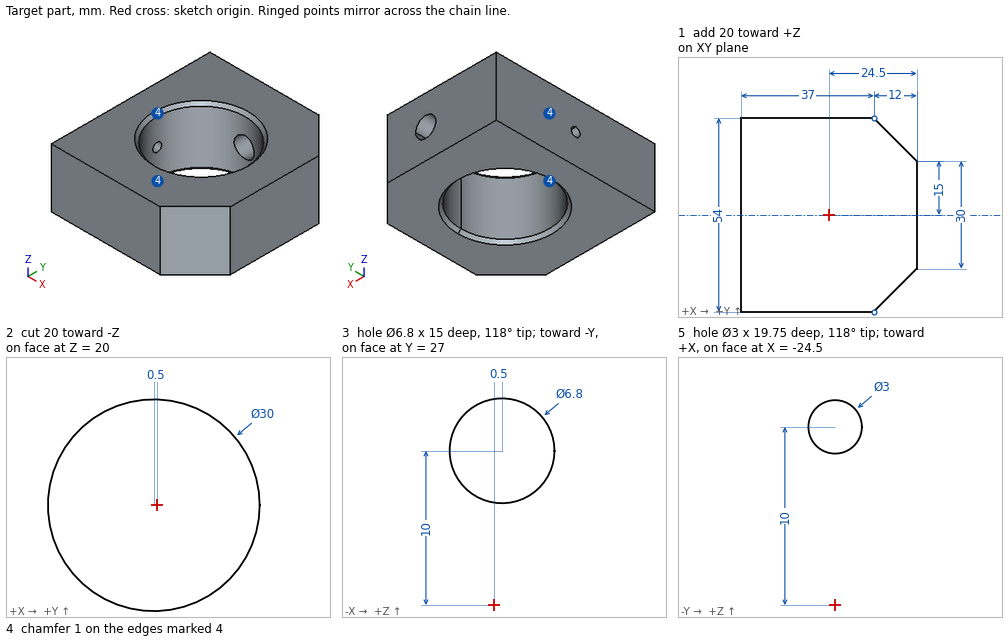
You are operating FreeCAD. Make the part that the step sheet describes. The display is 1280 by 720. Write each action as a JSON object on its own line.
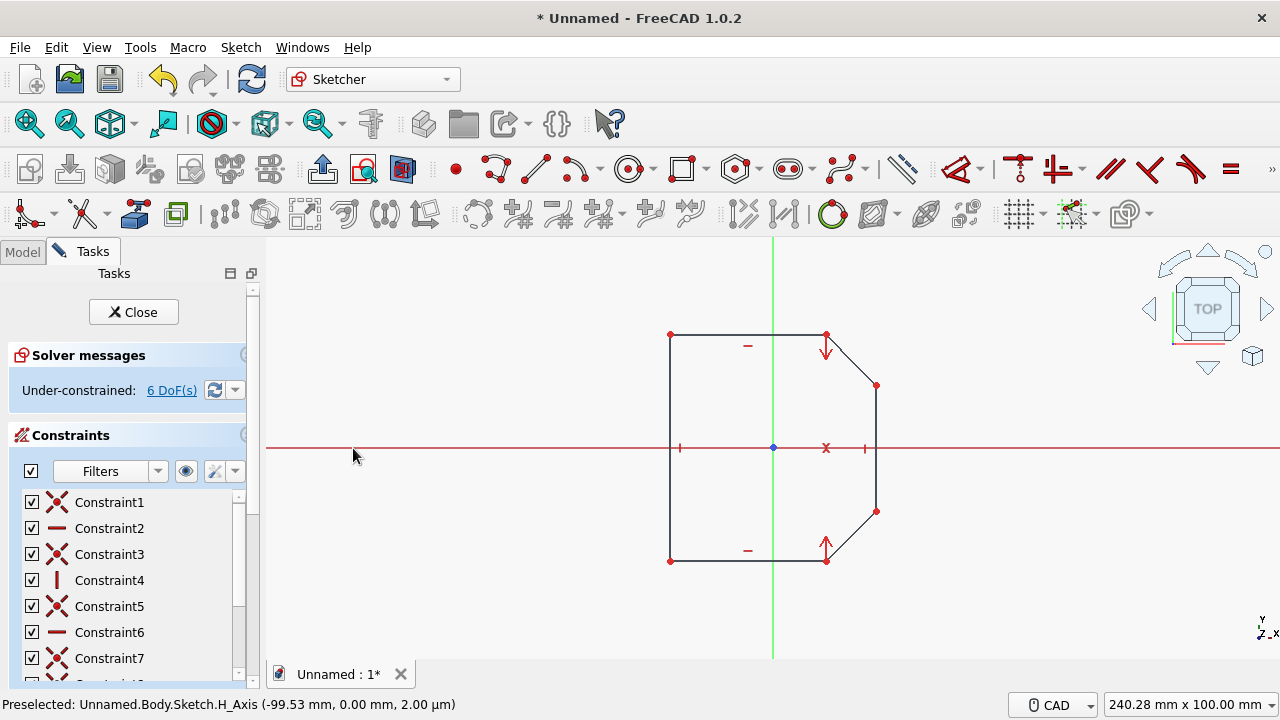
{"action": "left_click", "coordinate": [717, 335]}
{"action": "left_click", "coordinate": [748, 301]}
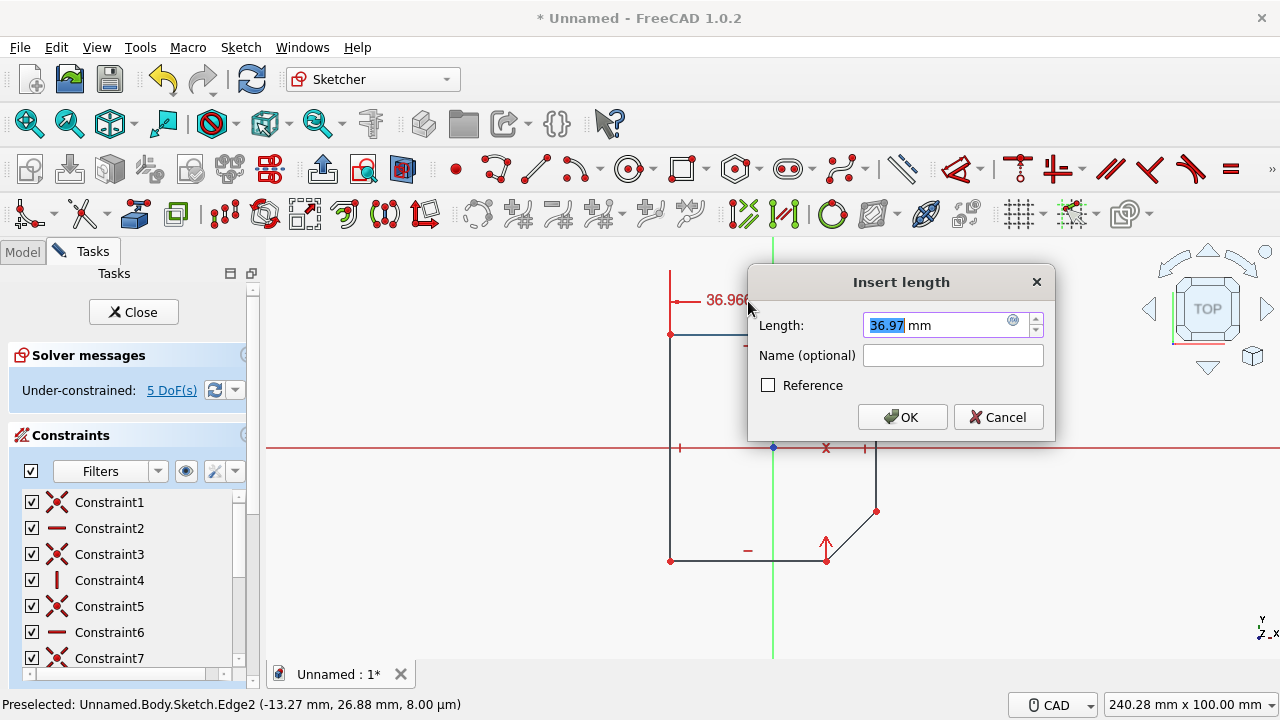
{"action": "type", "text": "37"}
{"action": "key", "text": "Return"}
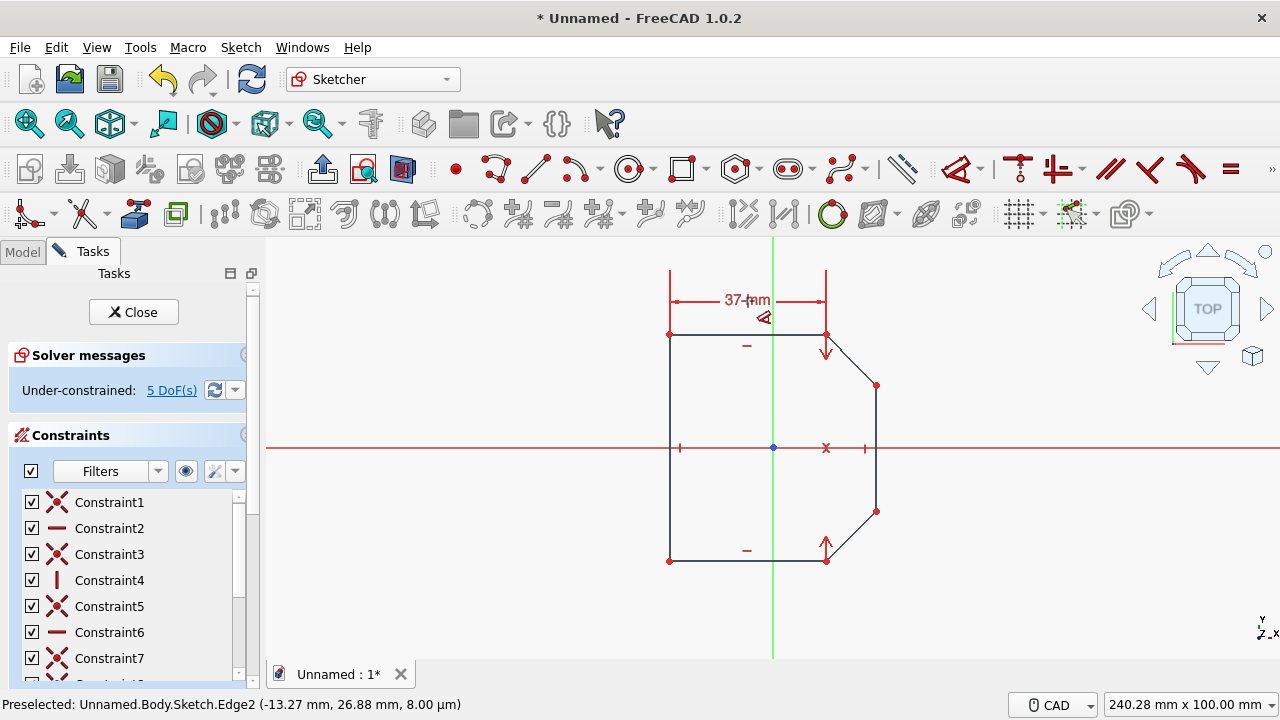
{"action": "left_click", "coordinate": [670, 403]}
{"action": "left_click", "coordinate": [636, 396]}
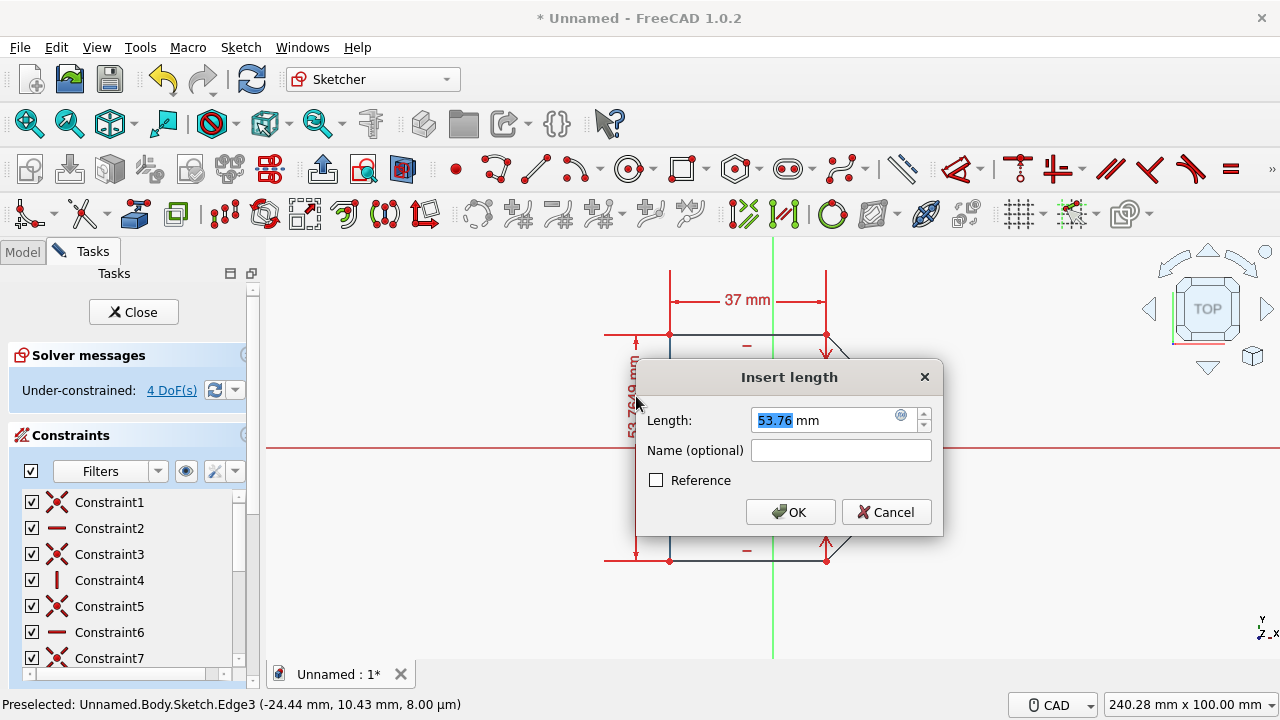
{"action": "type", "text": "54"}
{"action": "key", "text": "Return"}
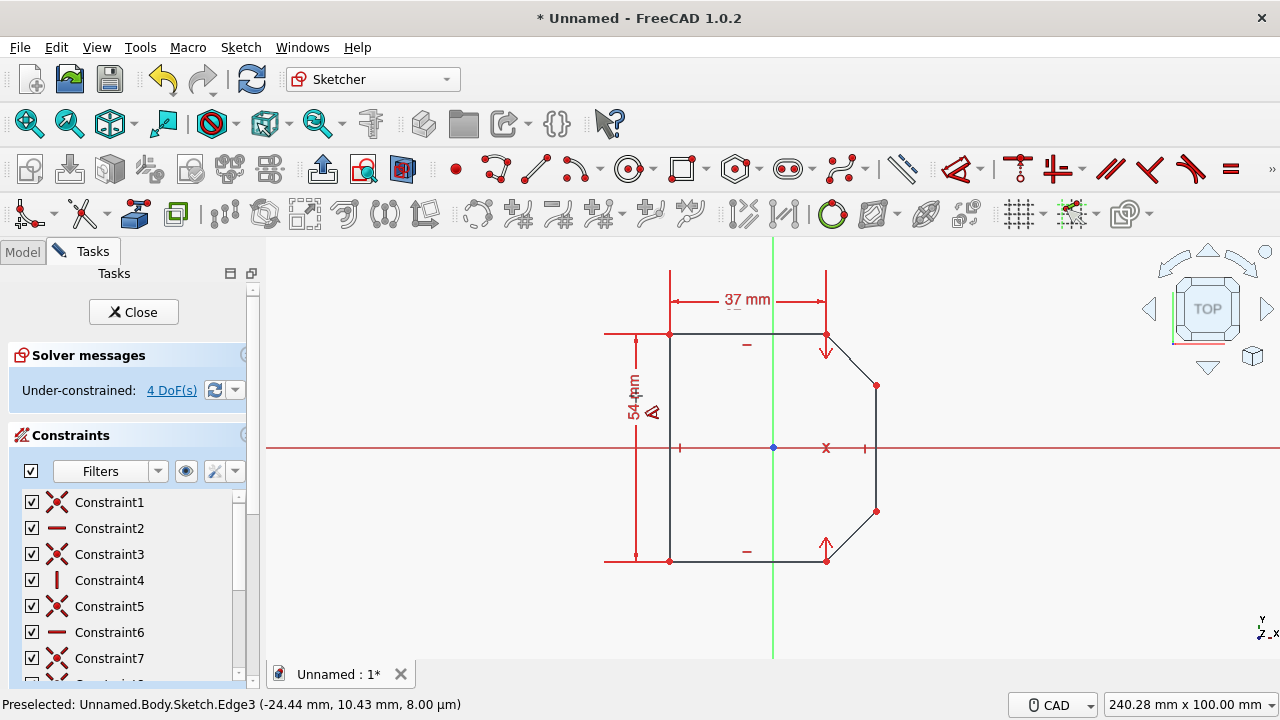
{"action": "left_click", "coordinate": [876, 474]}
{"action": "left_click", "coordinate": [910, 420]}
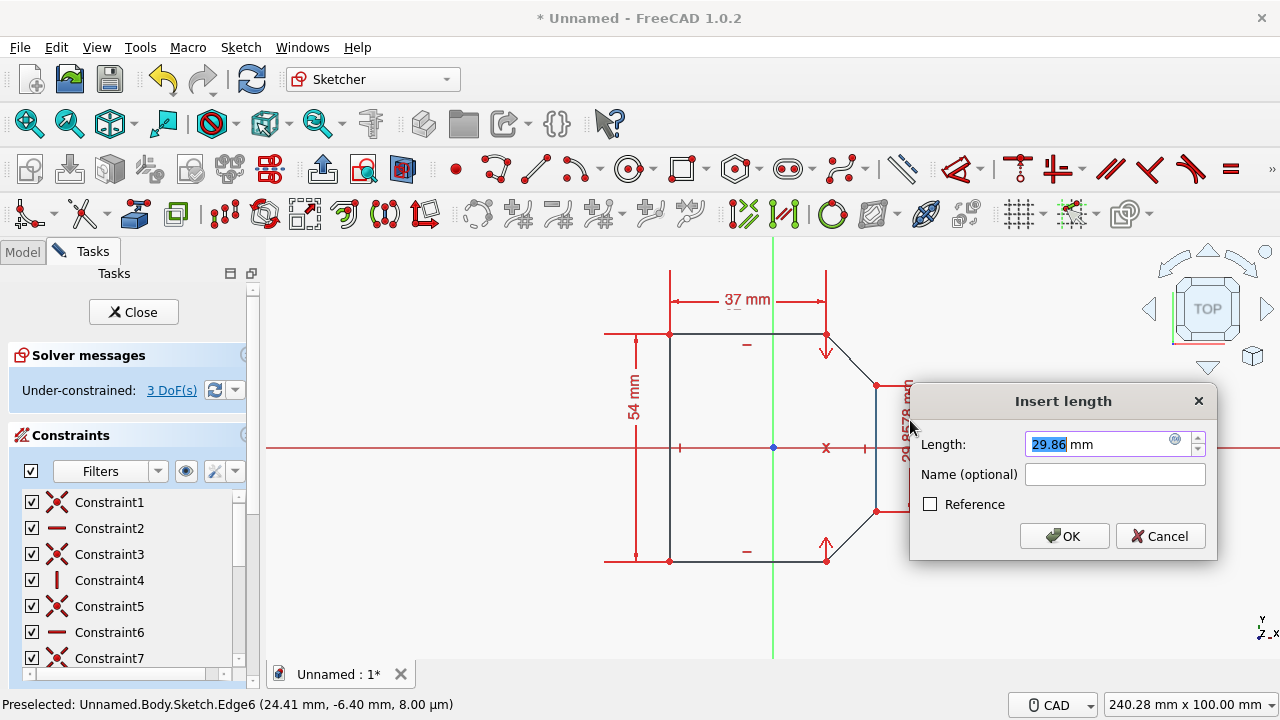
{"action": "type", "text": "30"}
{"action": "key", "text": "Return"}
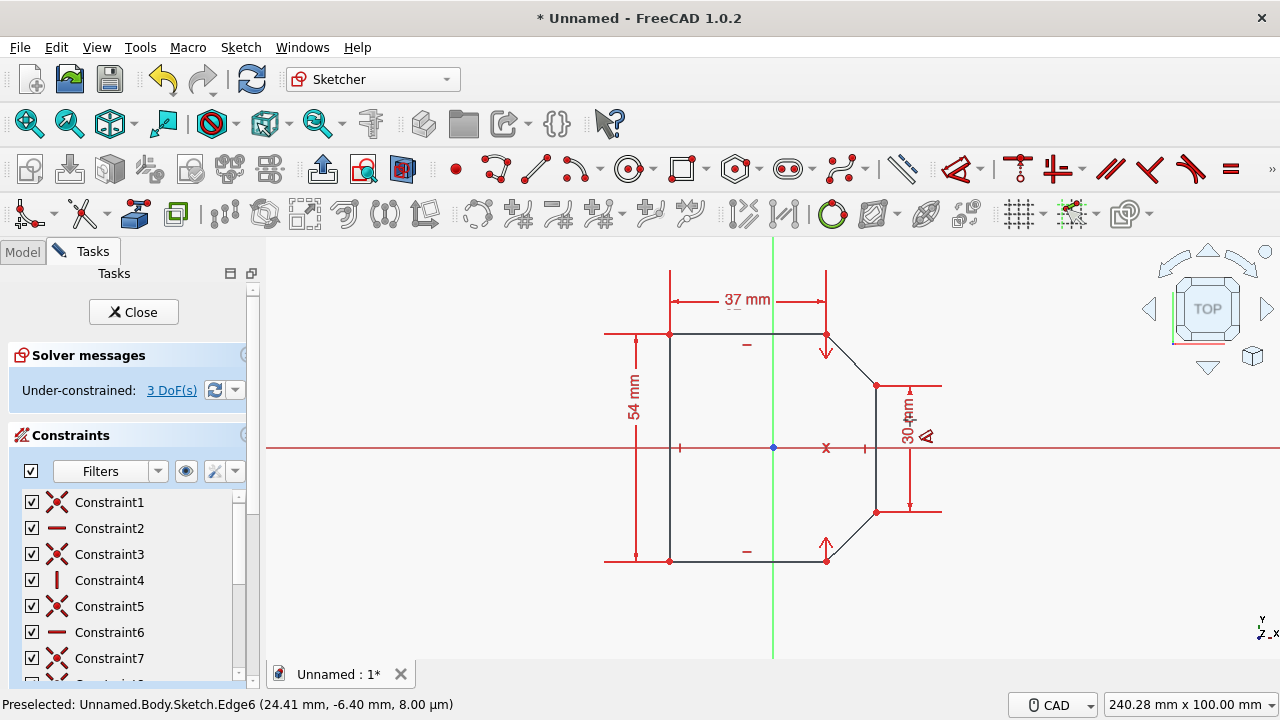
{"action": "left_click", "coordinate": [876, 386]}
{"action": "left_click", "coordinate": [910, 395]}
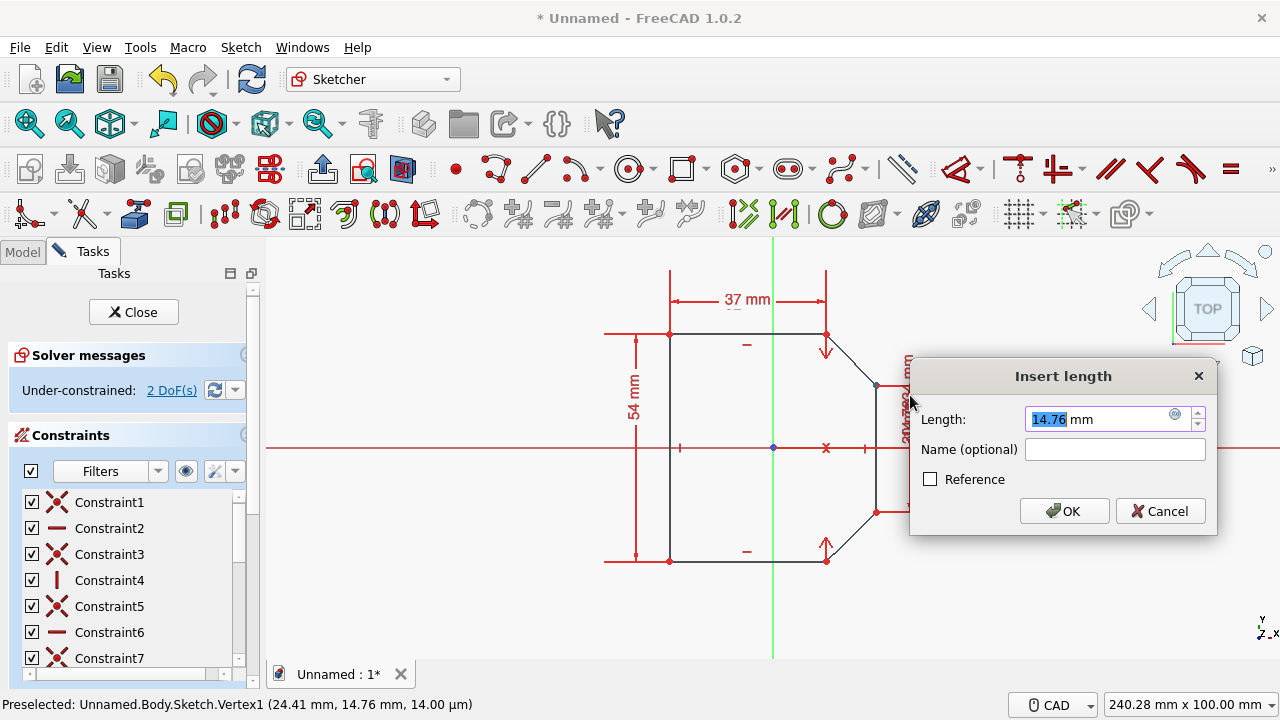
{"action": "type", "text": "15"}
{"action": "key", "text": "Return"}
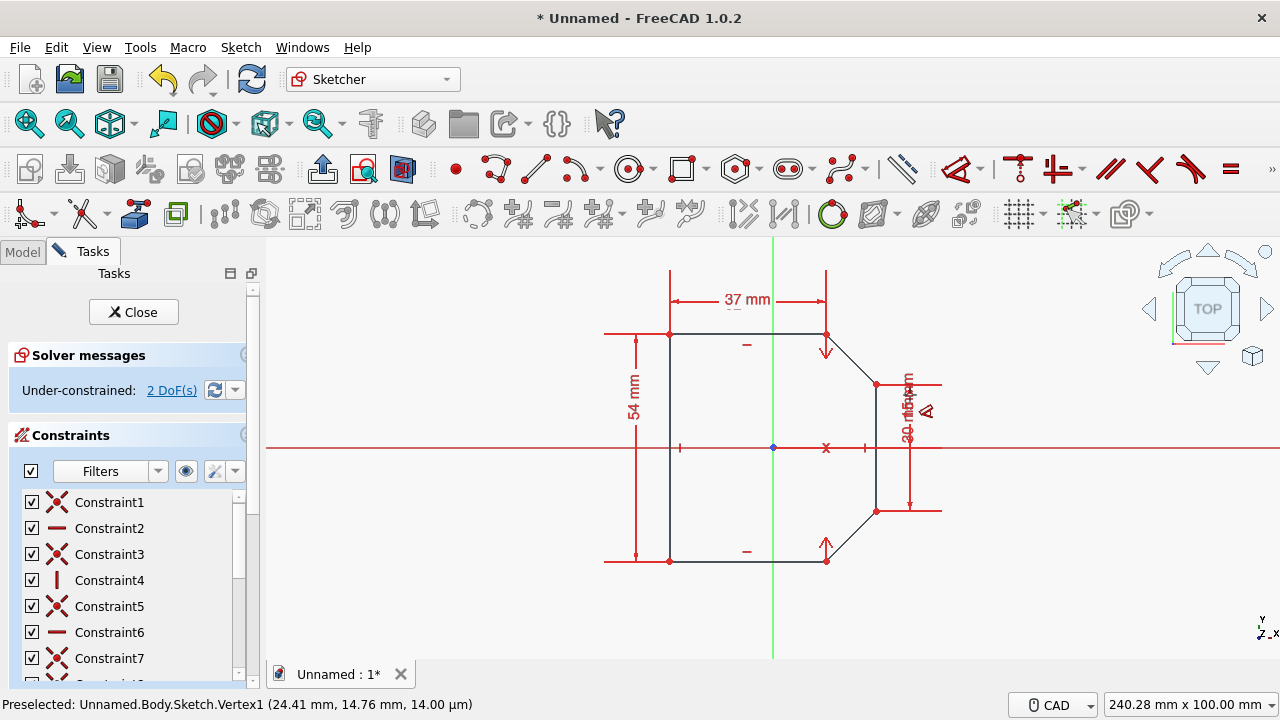
{"action": "left_click", "coordinate": [861, 370]}
{"action": "left_click", "coordinate": [851, 300]}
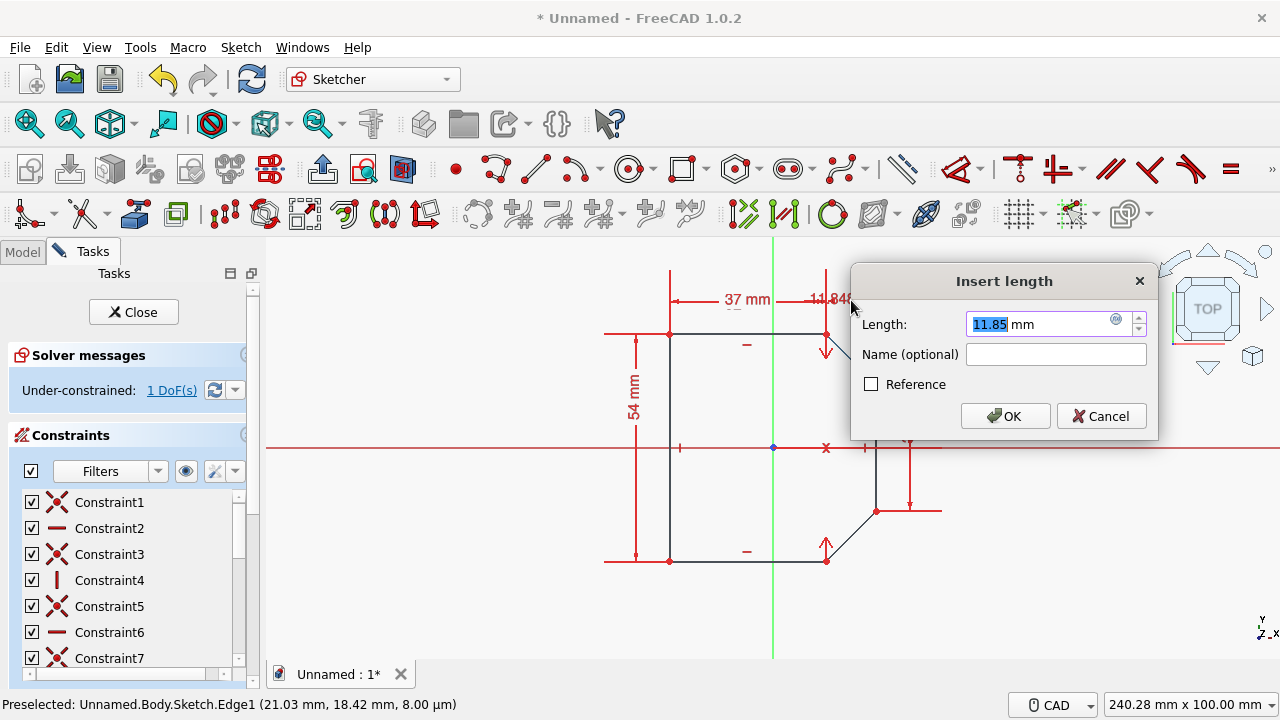
{"action": "type", "text": "12"}
{"action": "key", "text": "Return"}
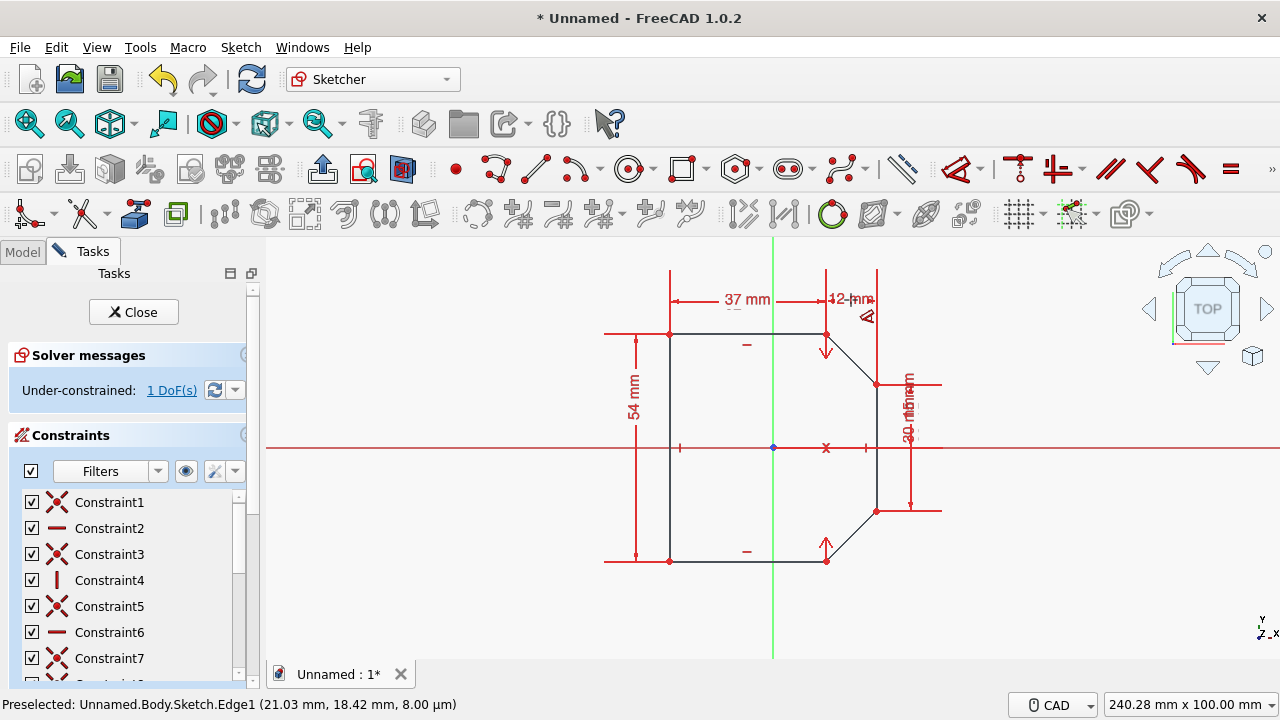
{"action": "left_click", "coordinate": [877, 385]}
{"action": "left_click", "coordinate": [801, 351]}